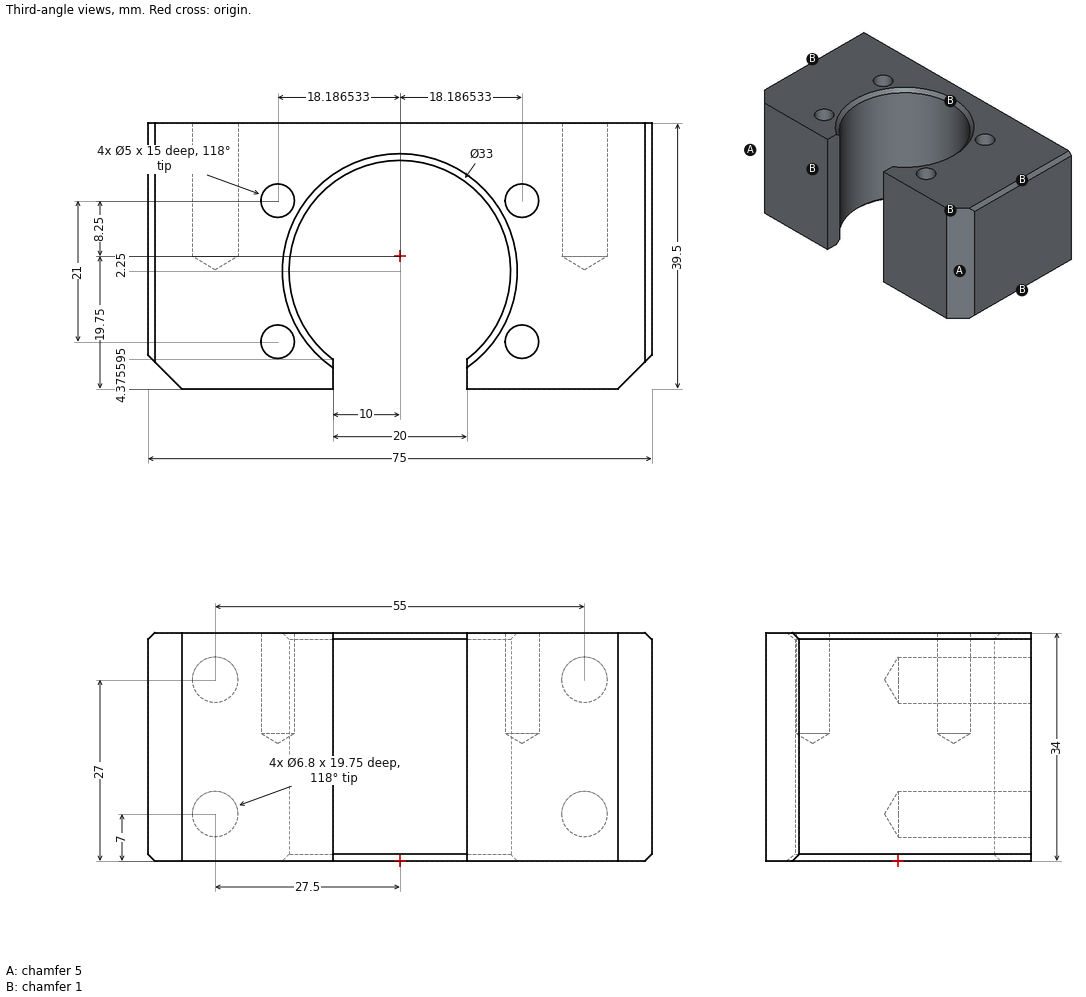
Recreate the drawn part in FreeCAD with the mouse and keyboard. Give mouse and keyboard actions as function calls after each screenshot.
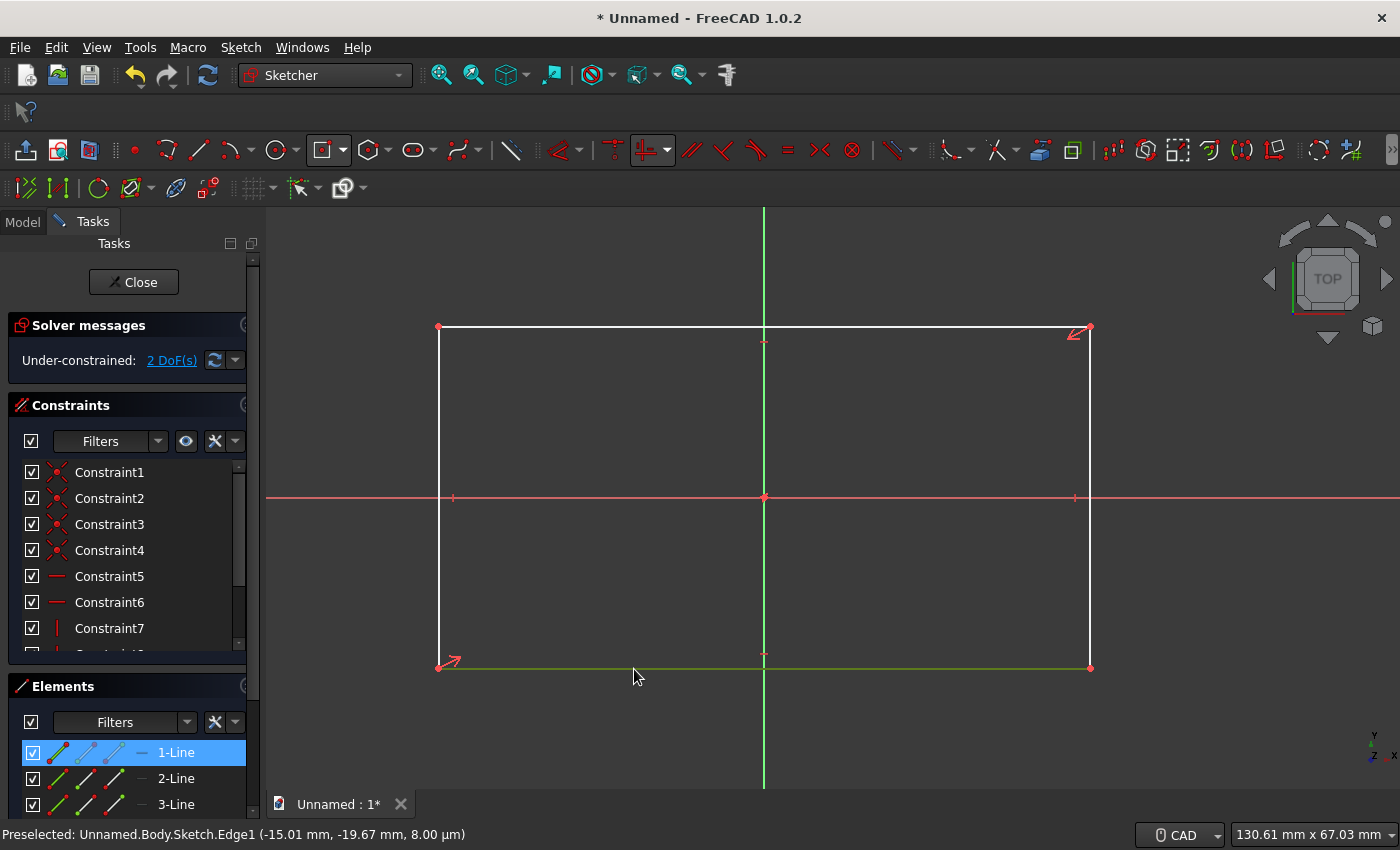
click(582, 150)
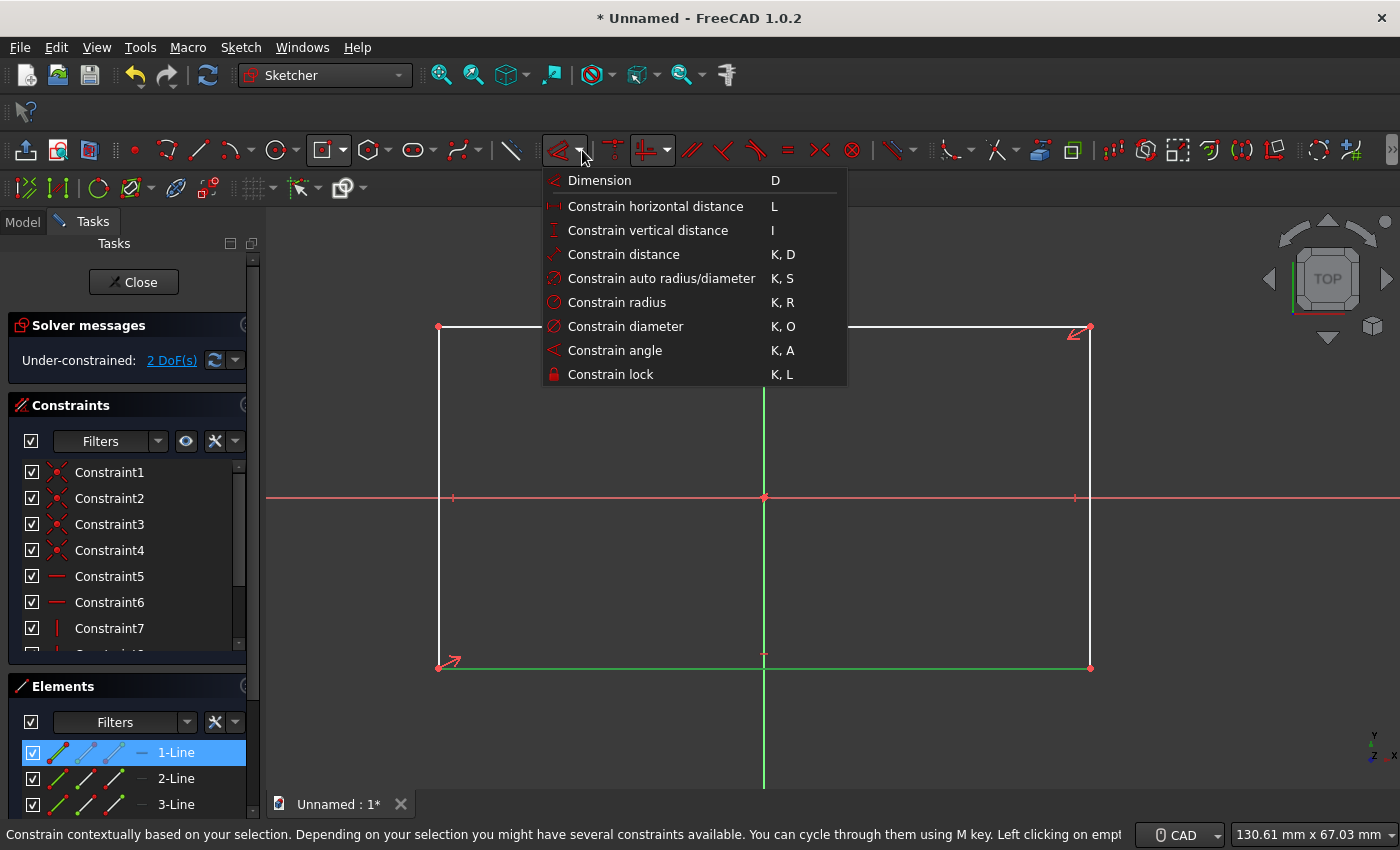
click(695, 206)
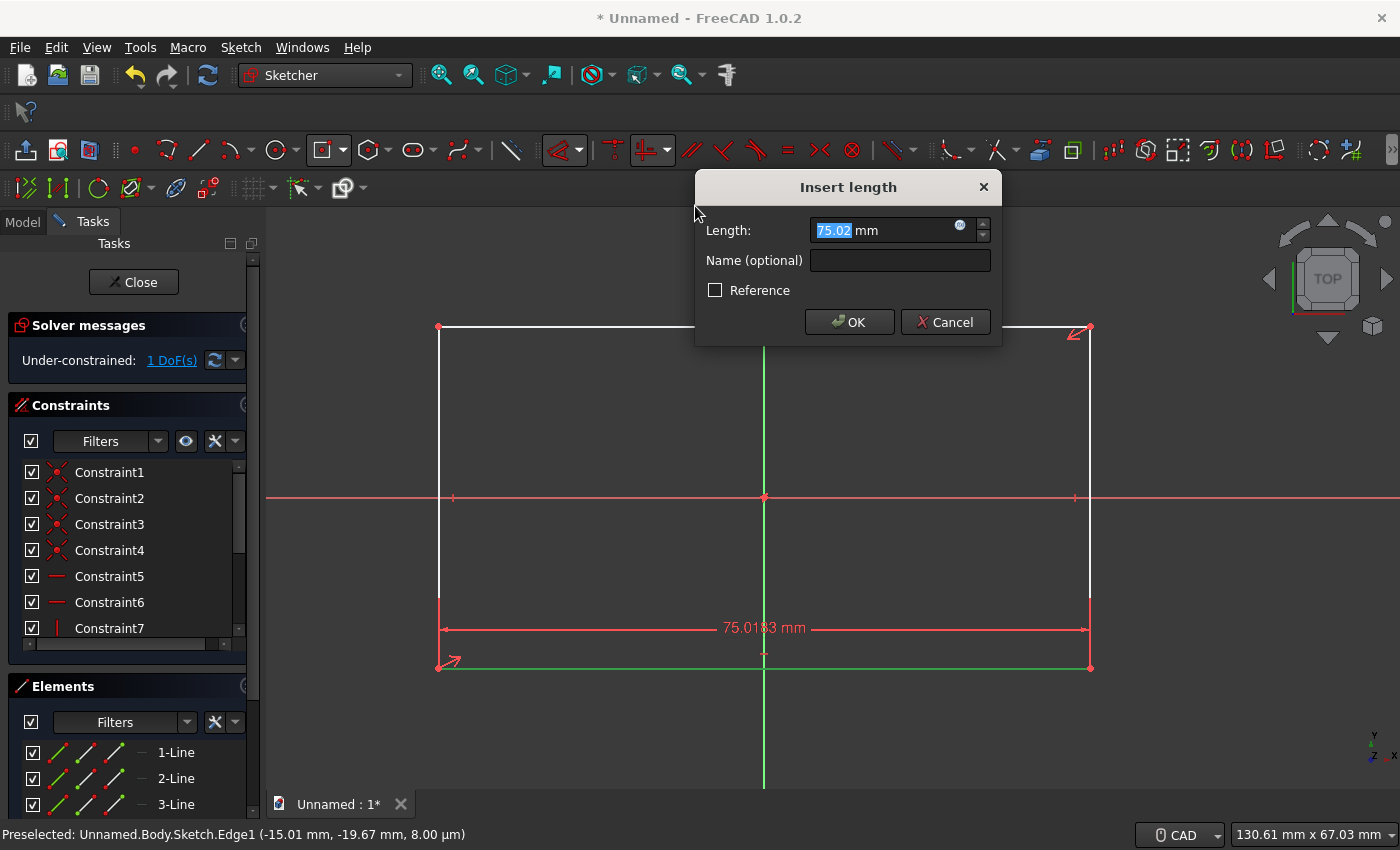
text(75)
key(Return)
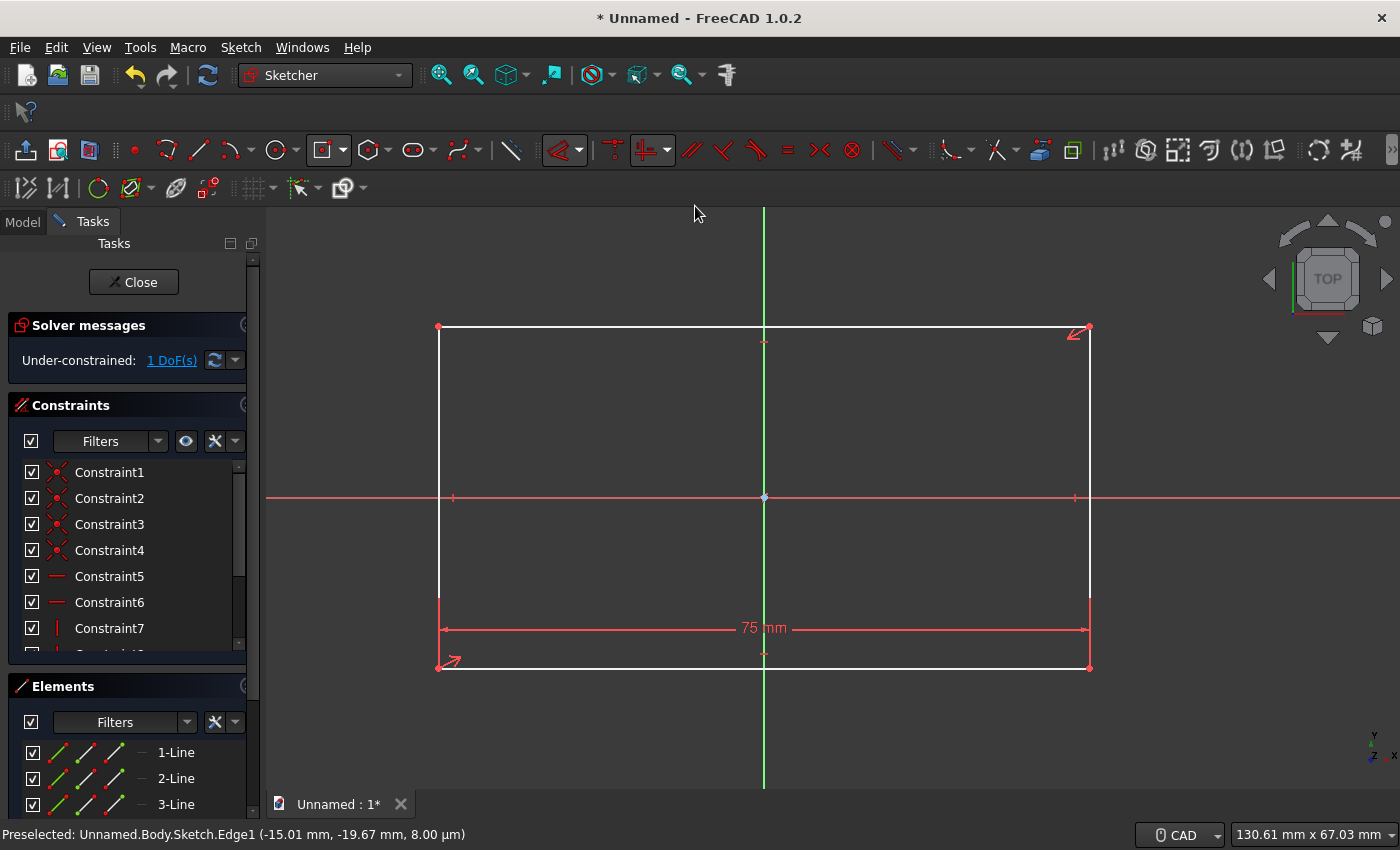
click(1090, 566)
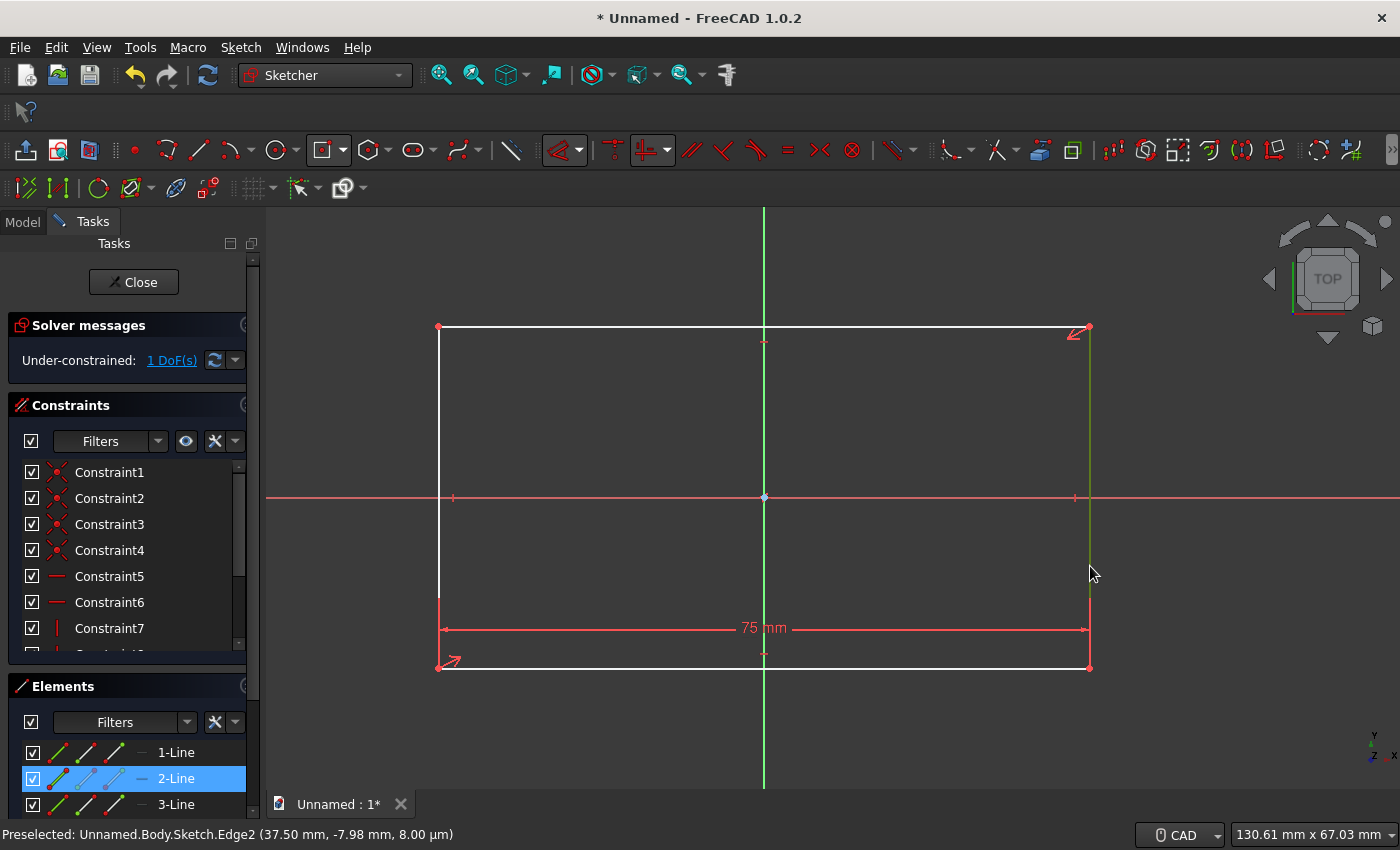
key(i)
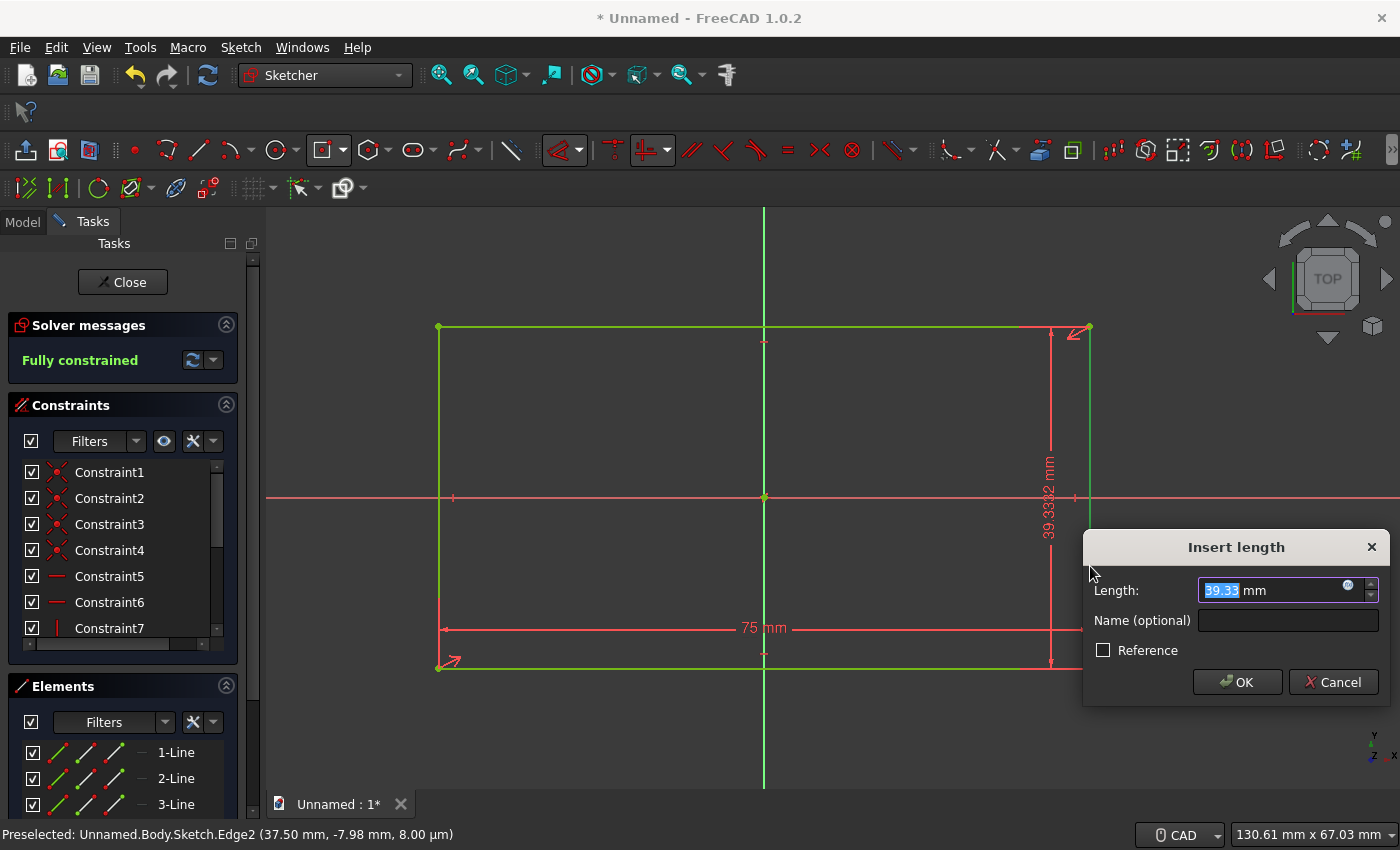
text(39.5)
key(Return)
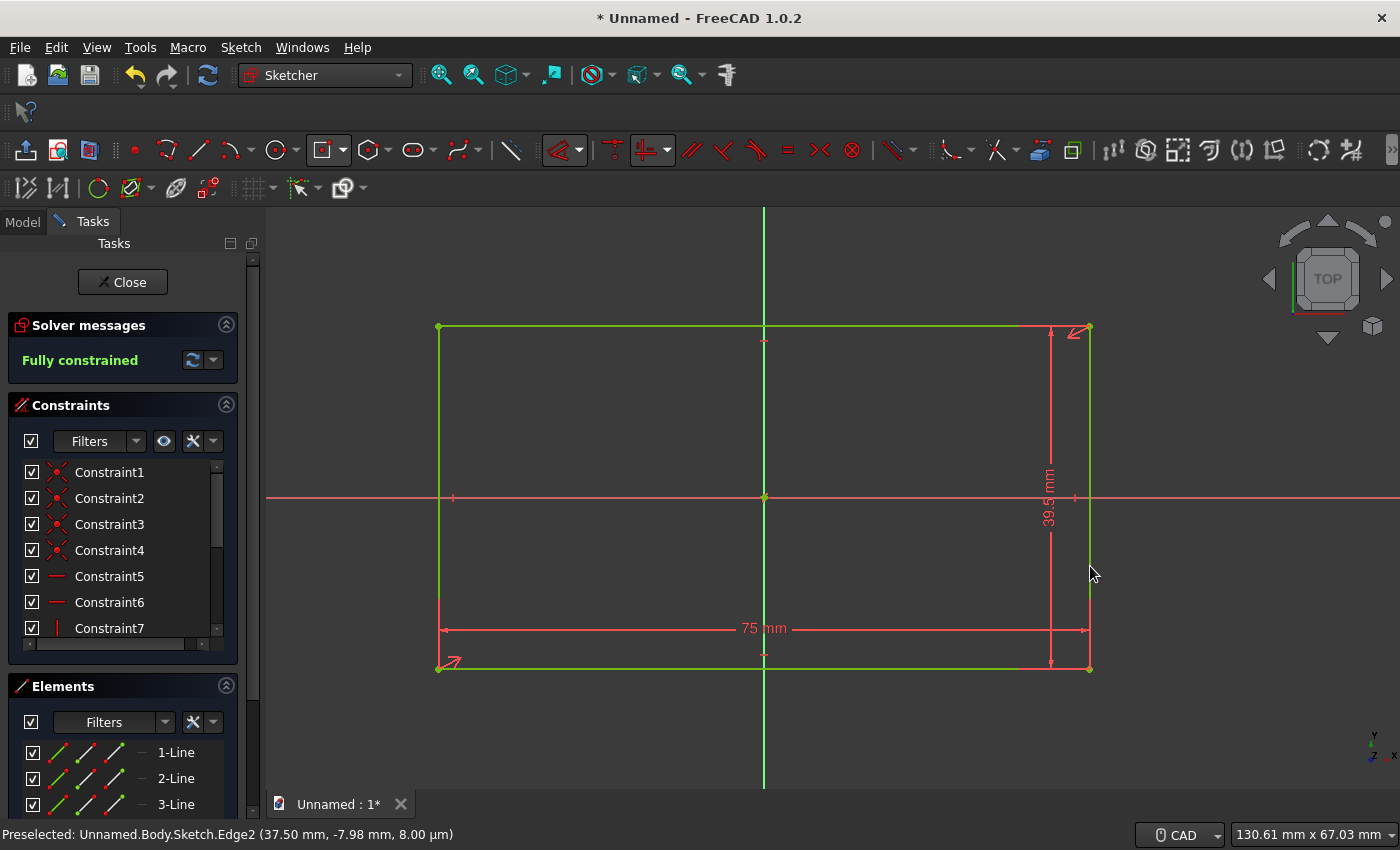
click(123, 282)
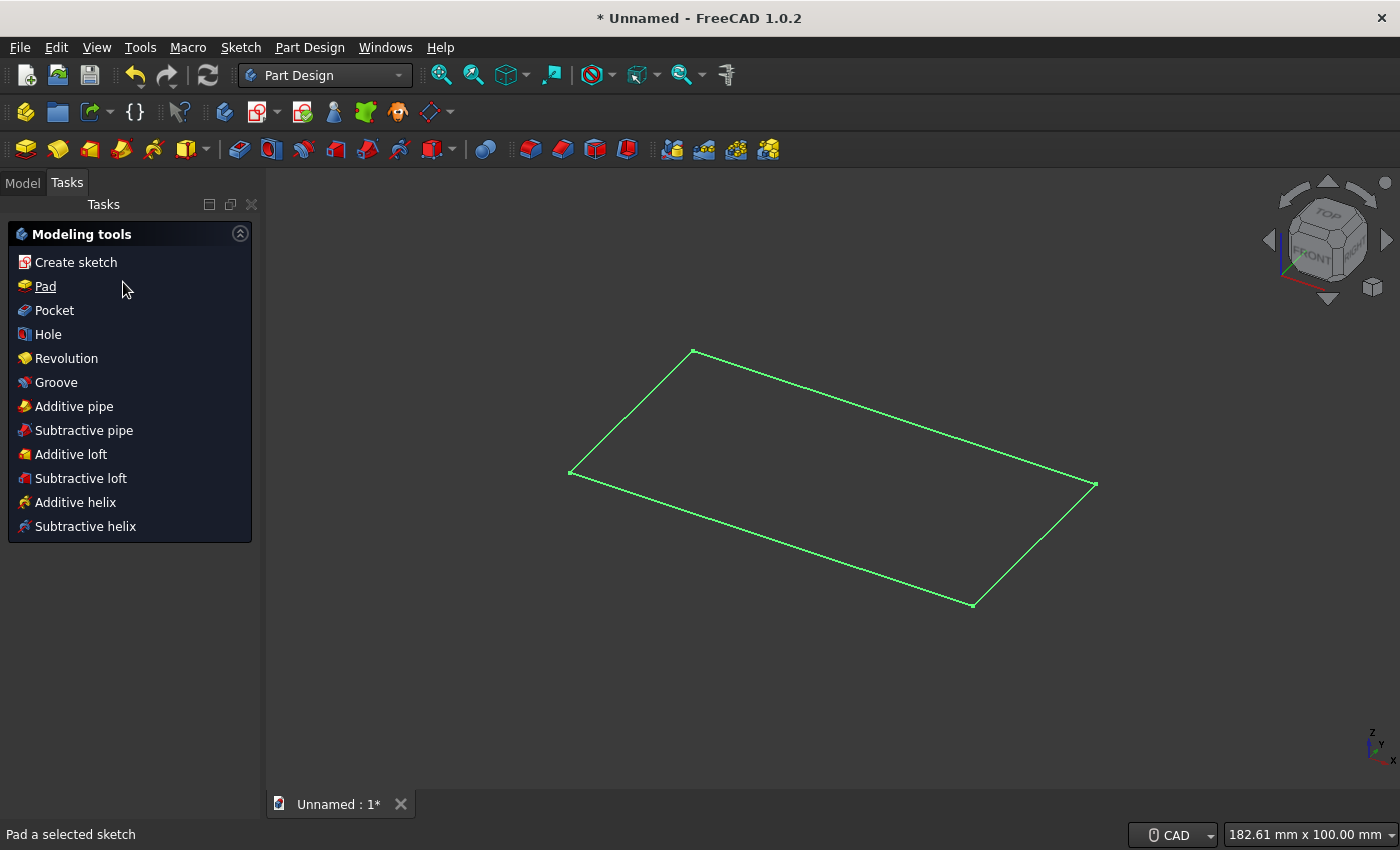
click(26, 150)